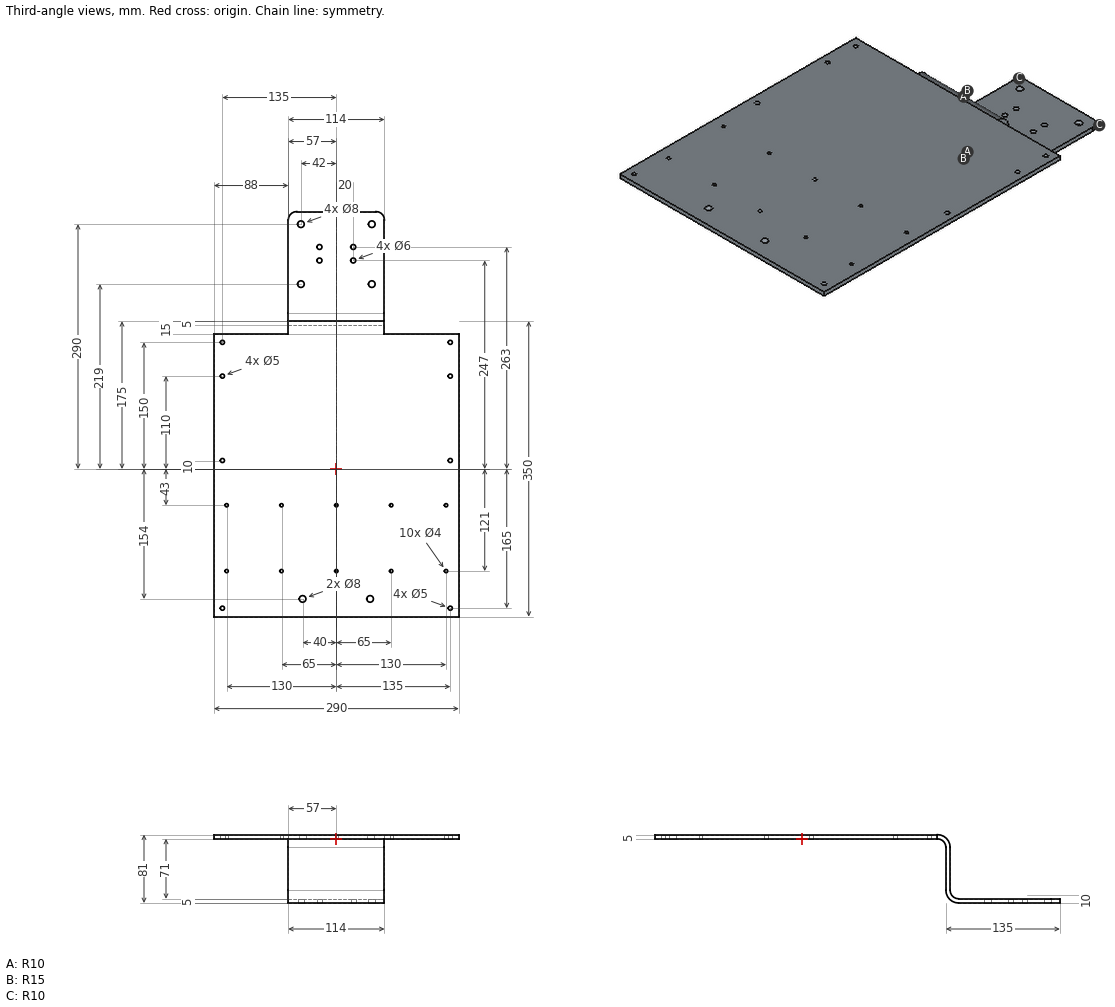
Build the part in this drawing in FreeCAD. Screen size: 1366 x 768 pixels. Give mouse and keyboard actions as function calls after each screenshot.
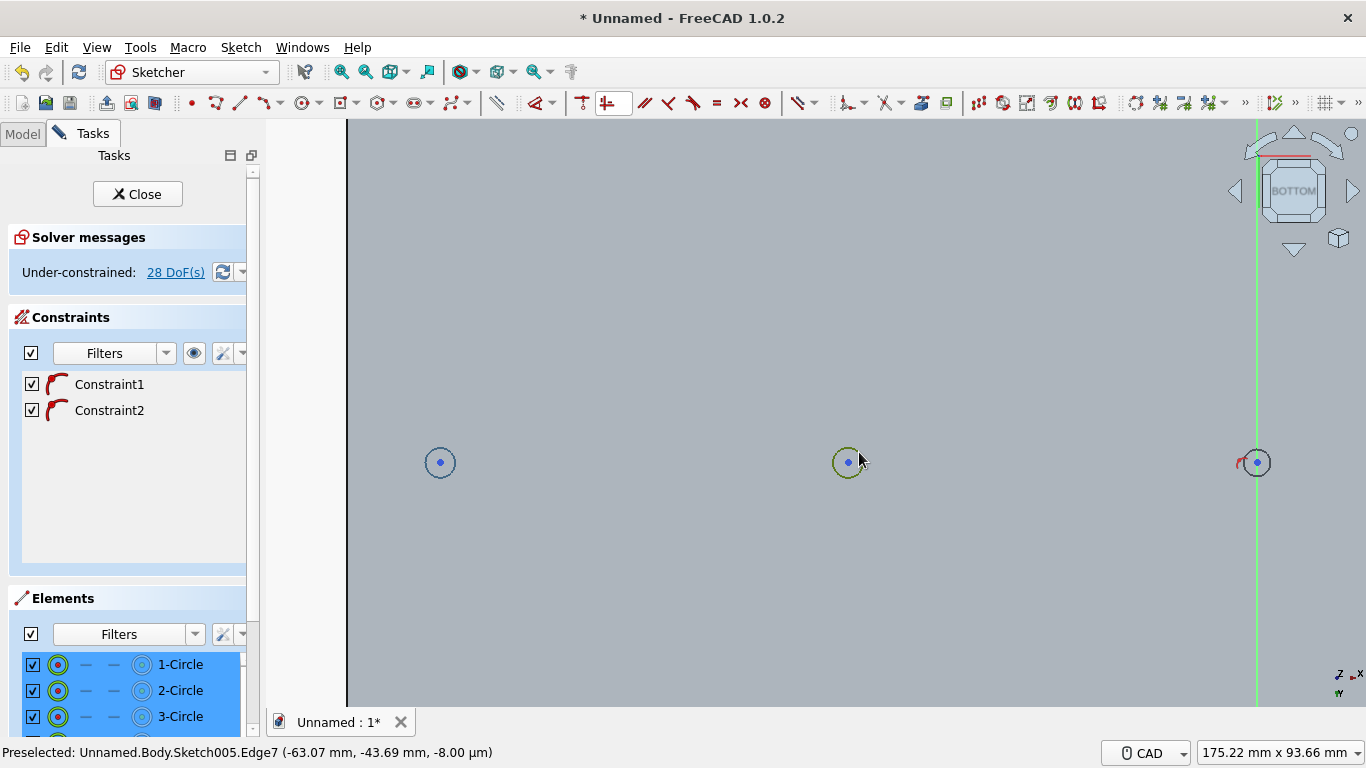
scroll(451, 453, down, 5)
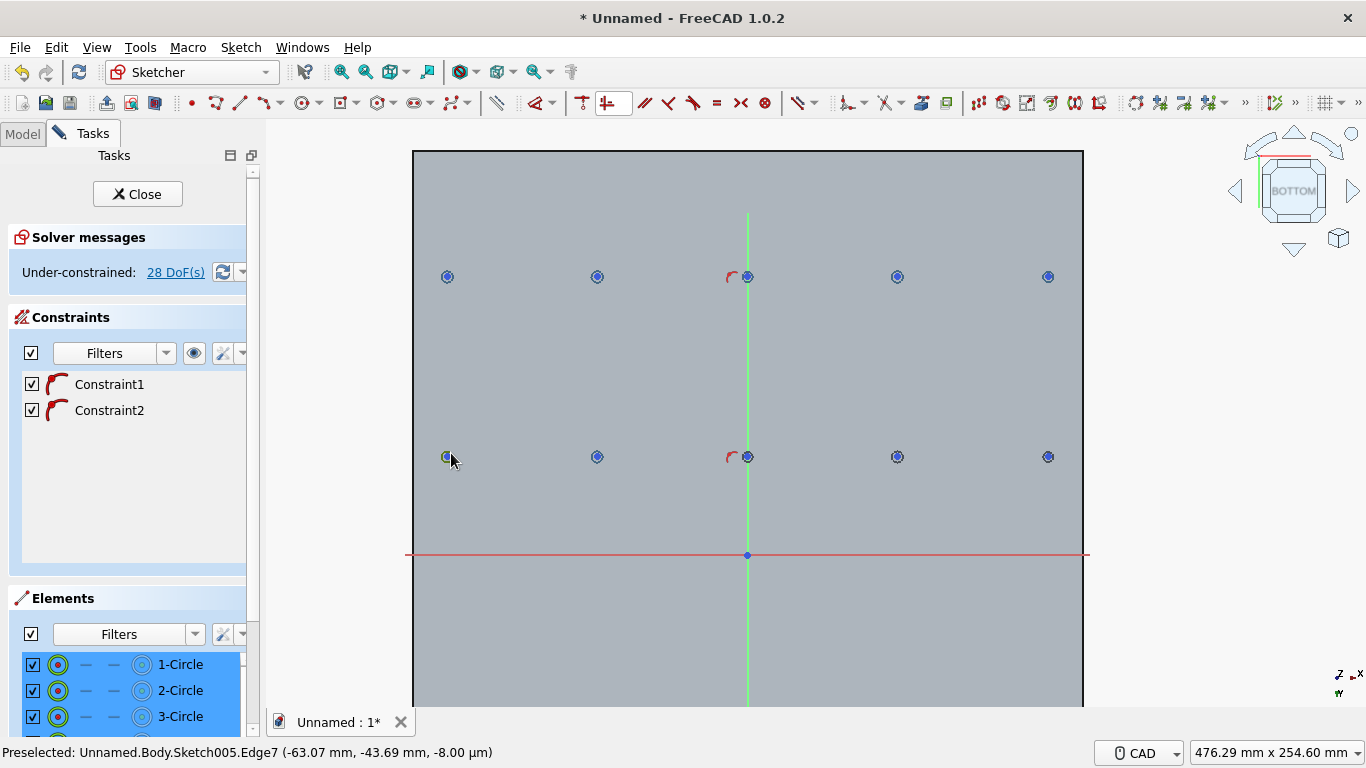
scroll(751, 454, up, 7)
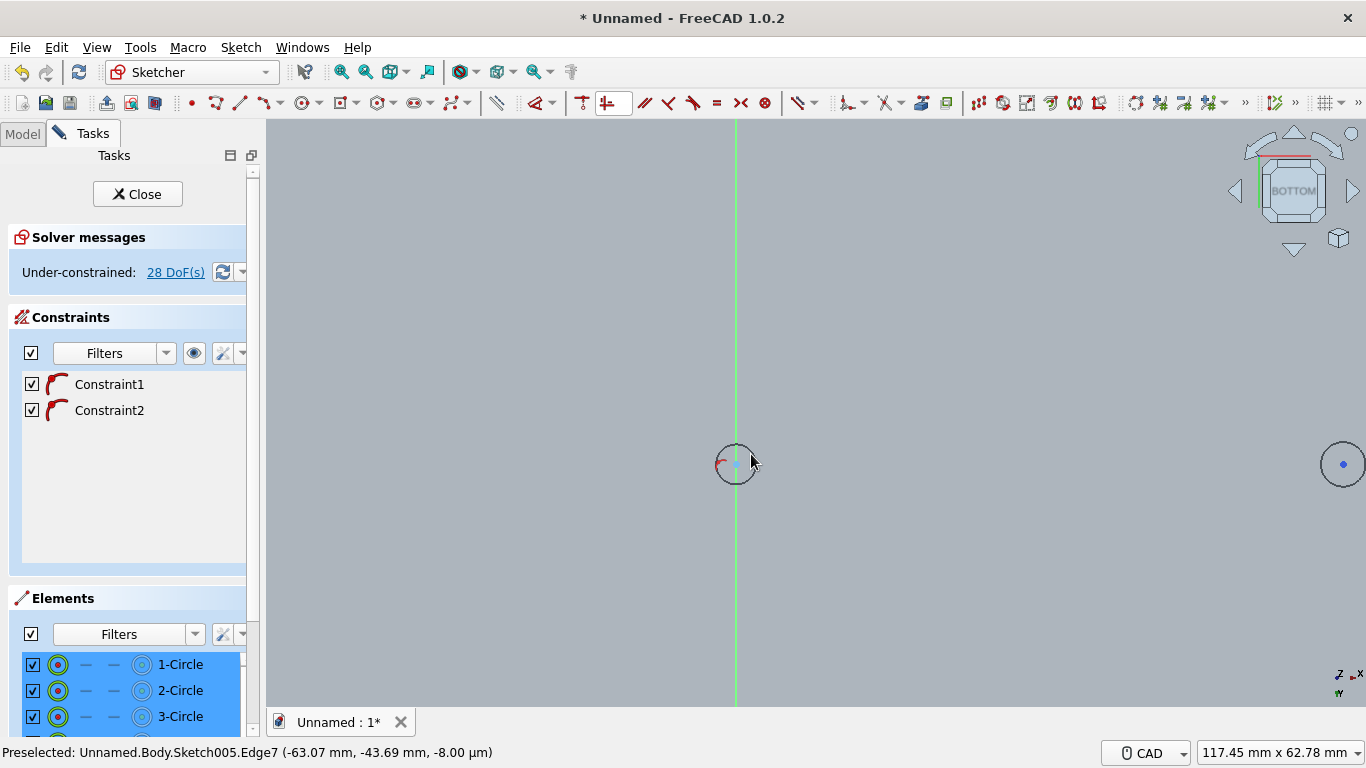
click(750, 450)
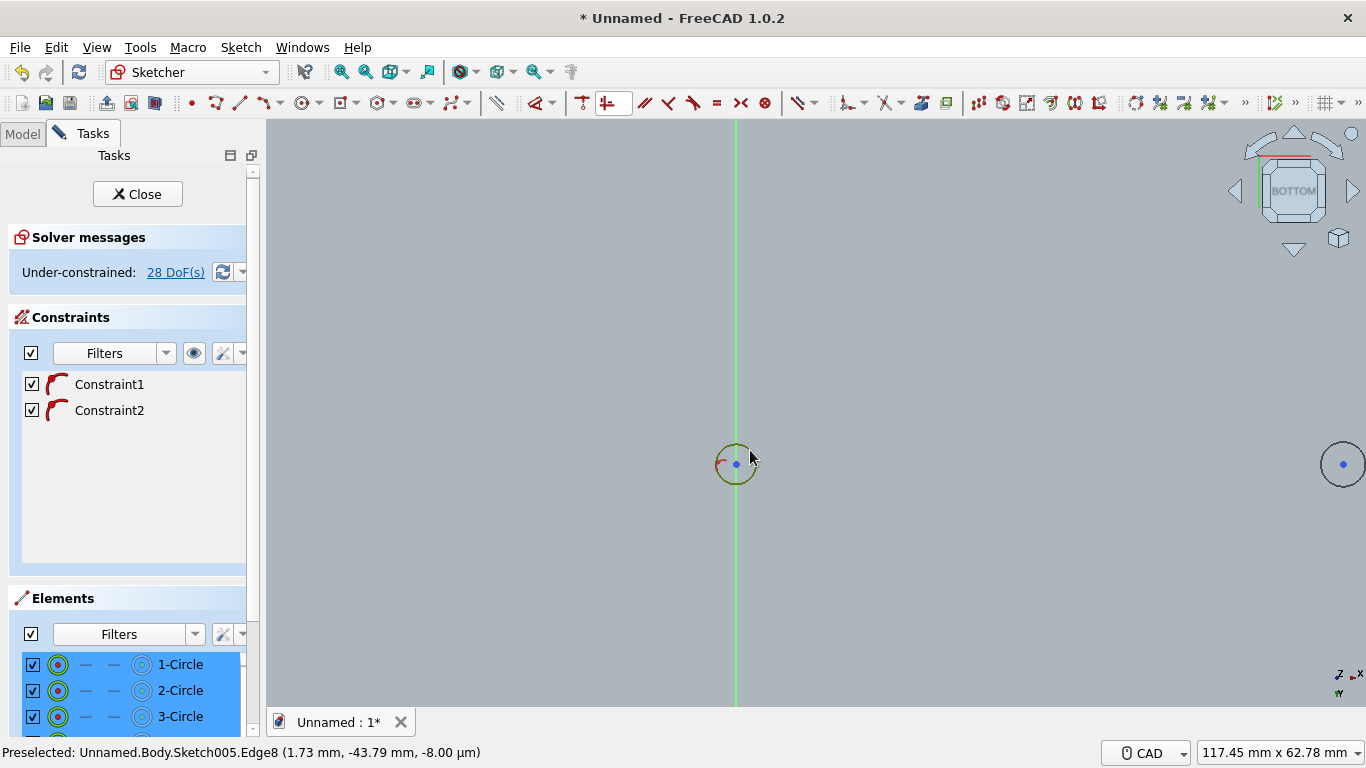
scroll(751, 454, down, 7)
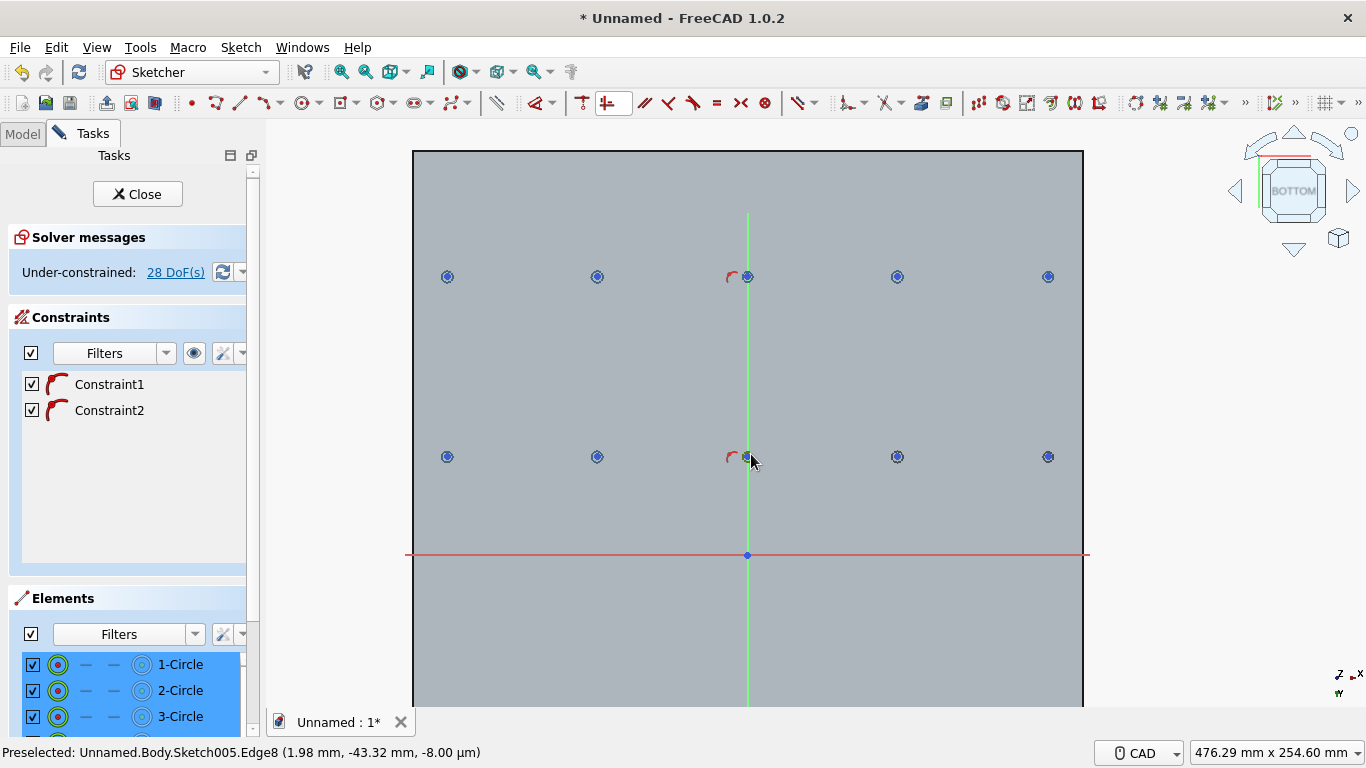
scroll(901, 453, up, 5)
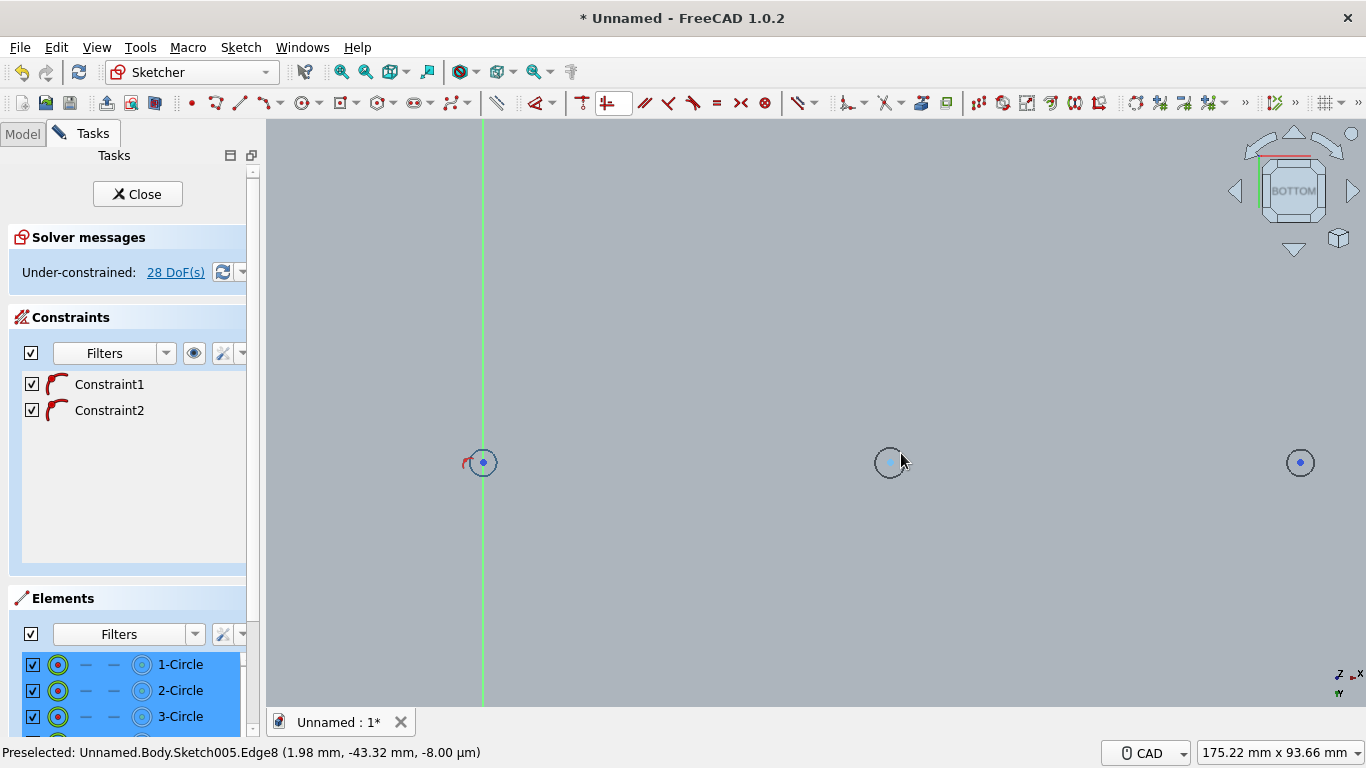
click(901, 452)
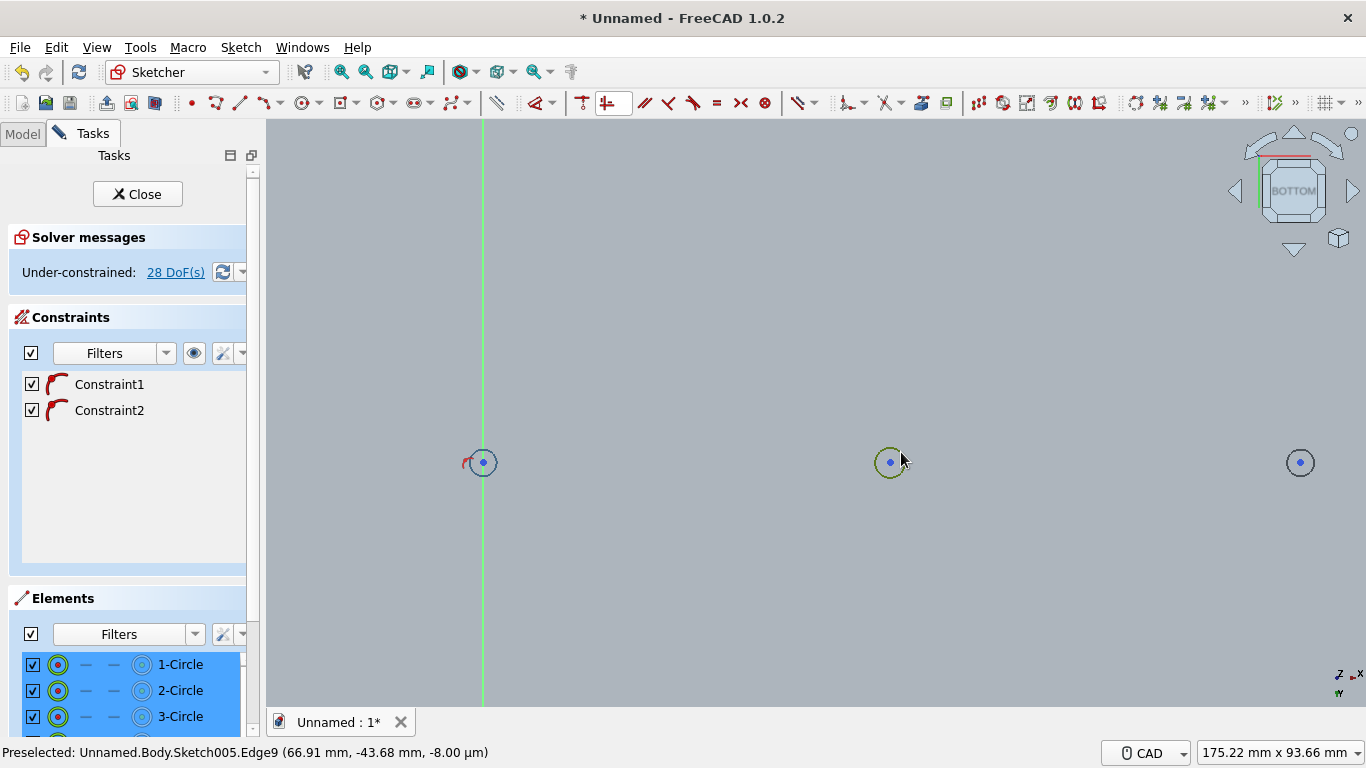
scroll(901, 453, down, 5)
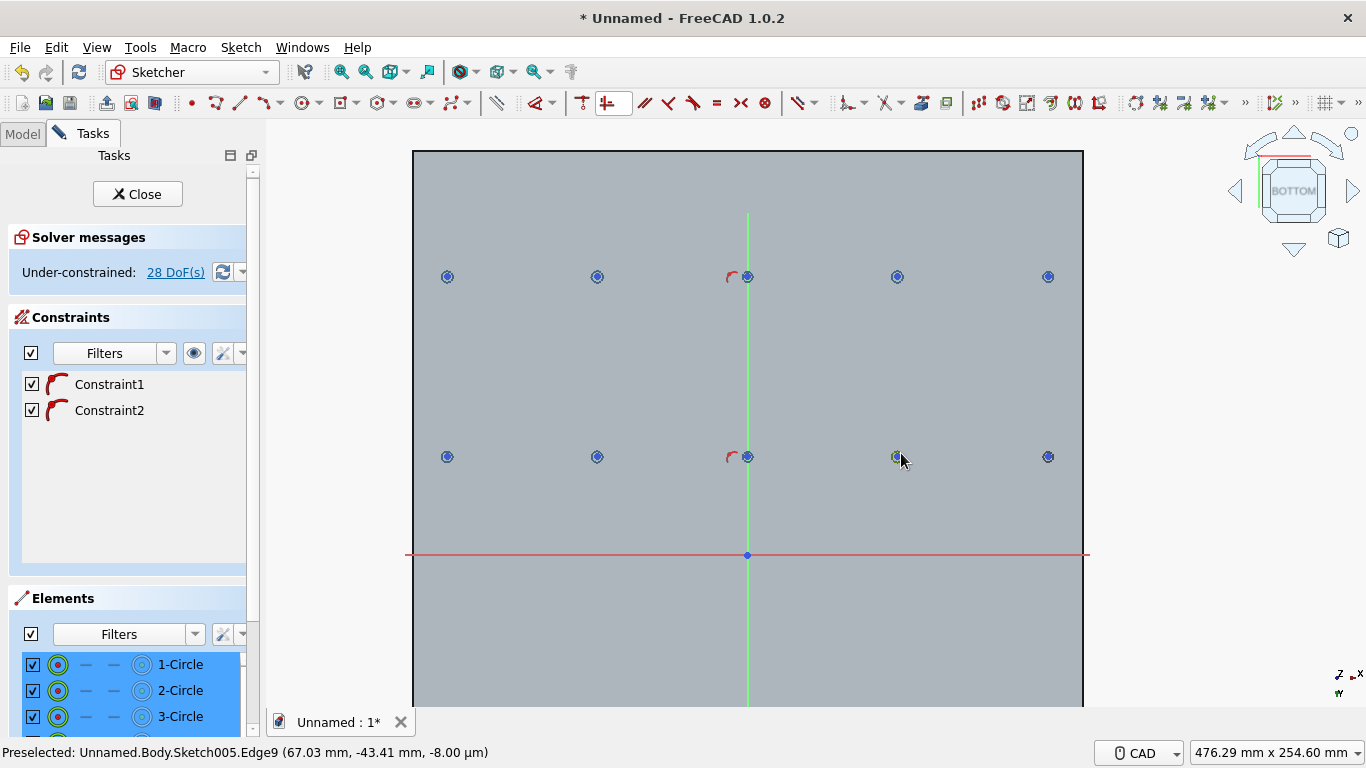
scroll(1052, 453, up, 6)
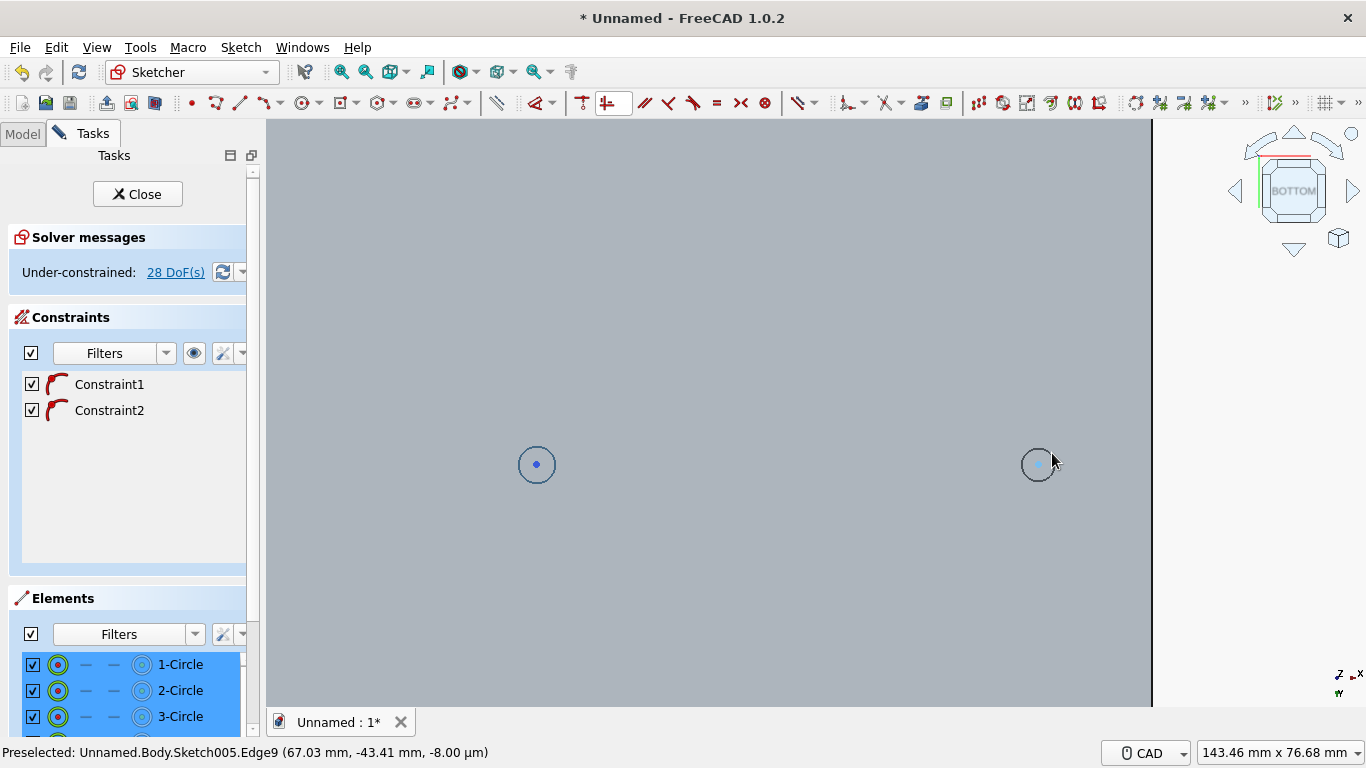
click(1050, 453)